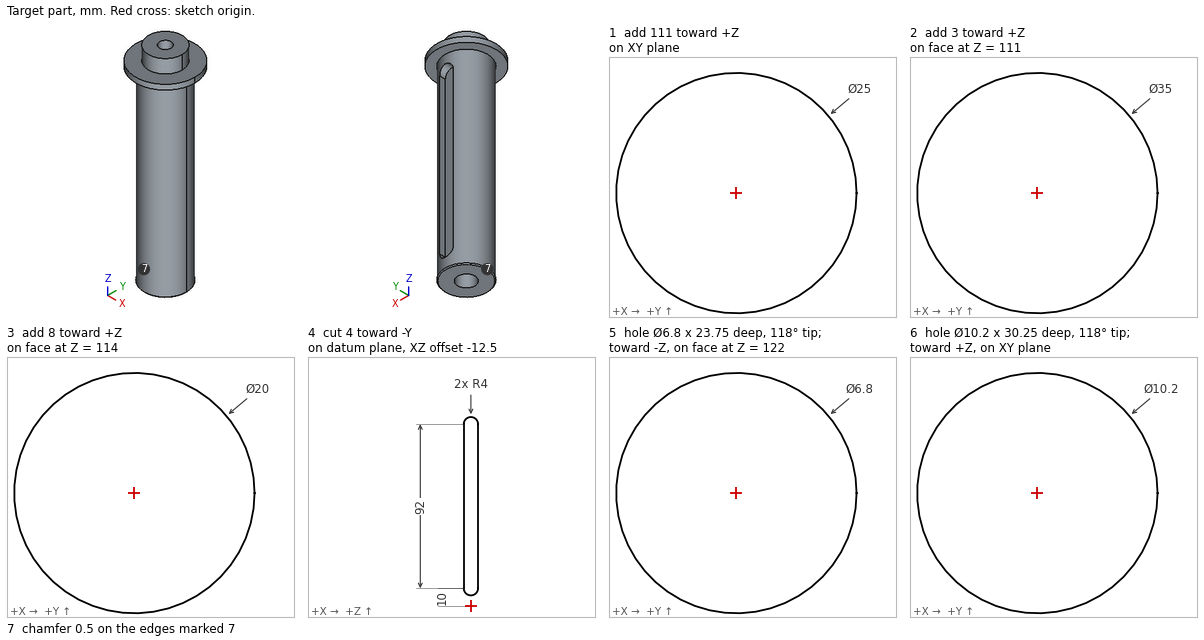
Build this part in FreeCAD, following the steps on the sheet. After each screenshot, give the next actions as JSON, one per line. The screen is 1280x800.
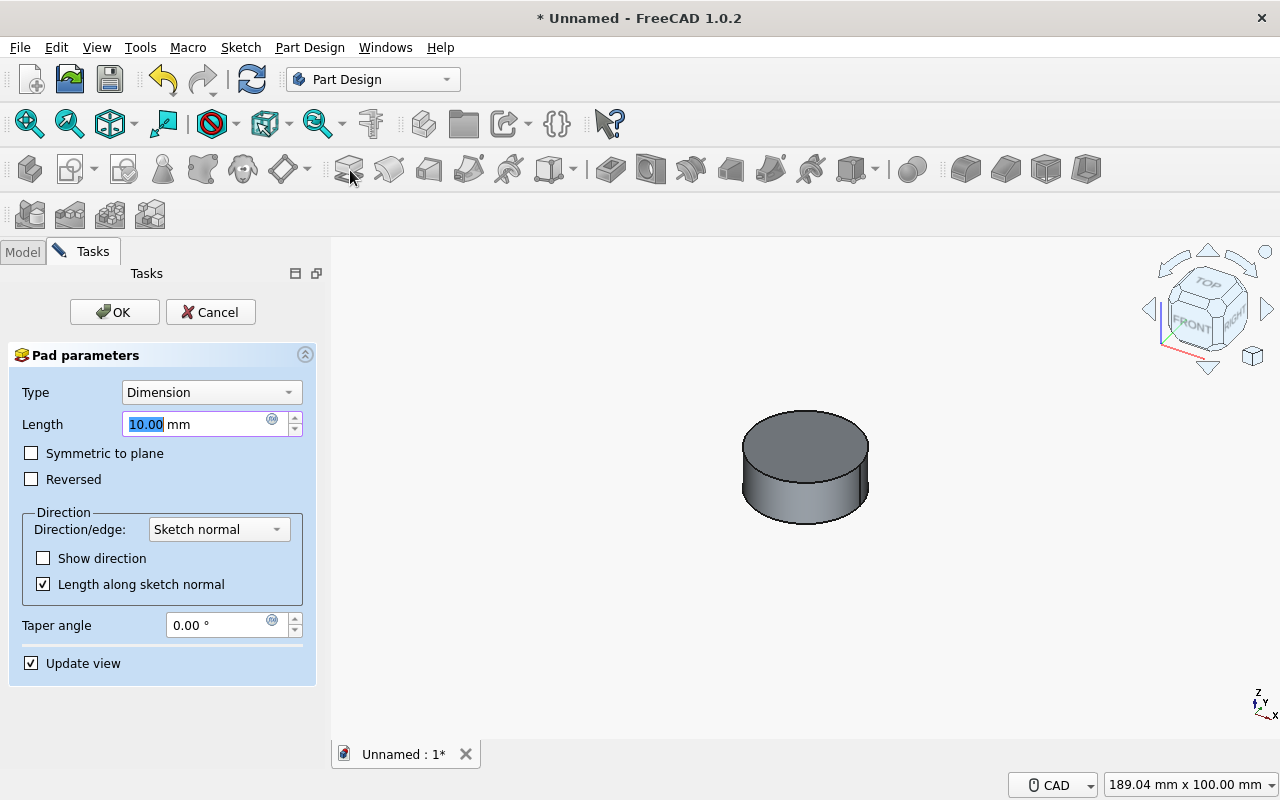
{"action": "type", "text": "111"}
{"action": "key", "text": "Tab"}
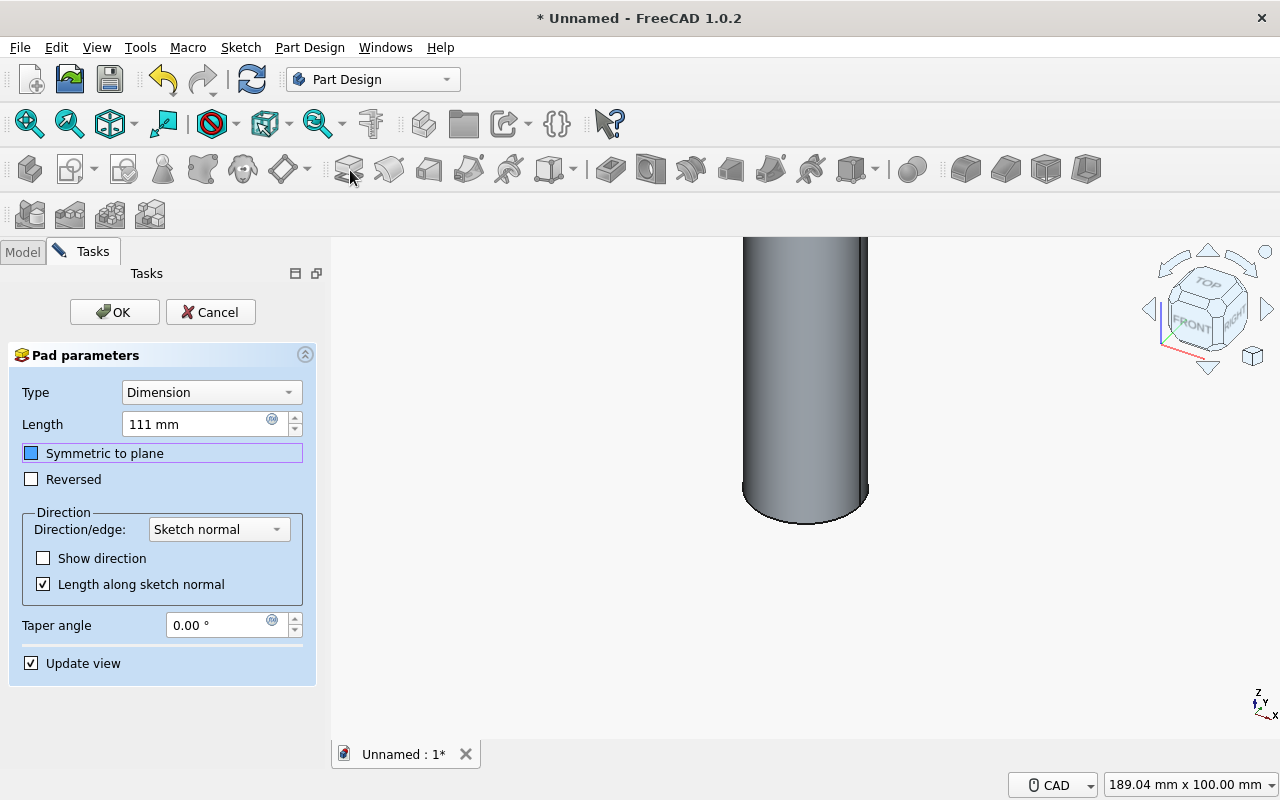
{"action": "left_click", "coordinate": [115, 312]}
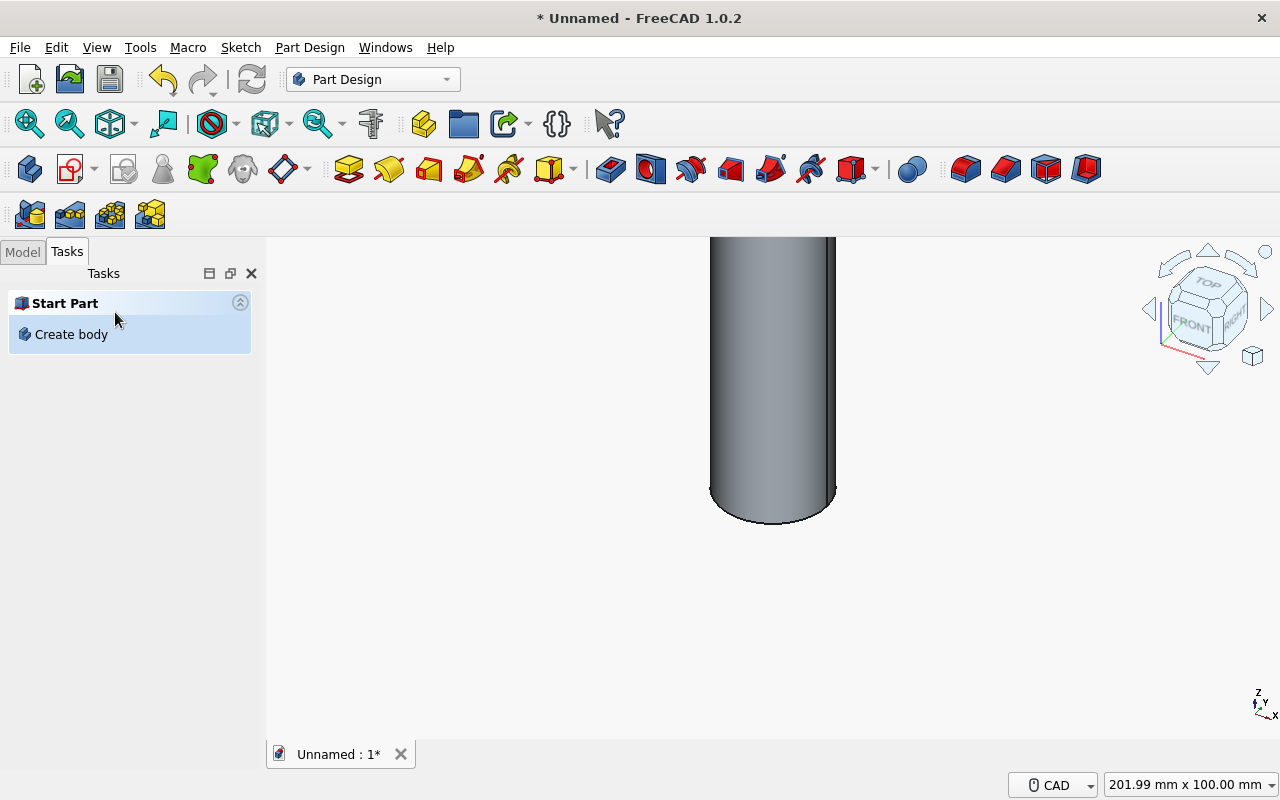
{"action": "key", "text": "v f"}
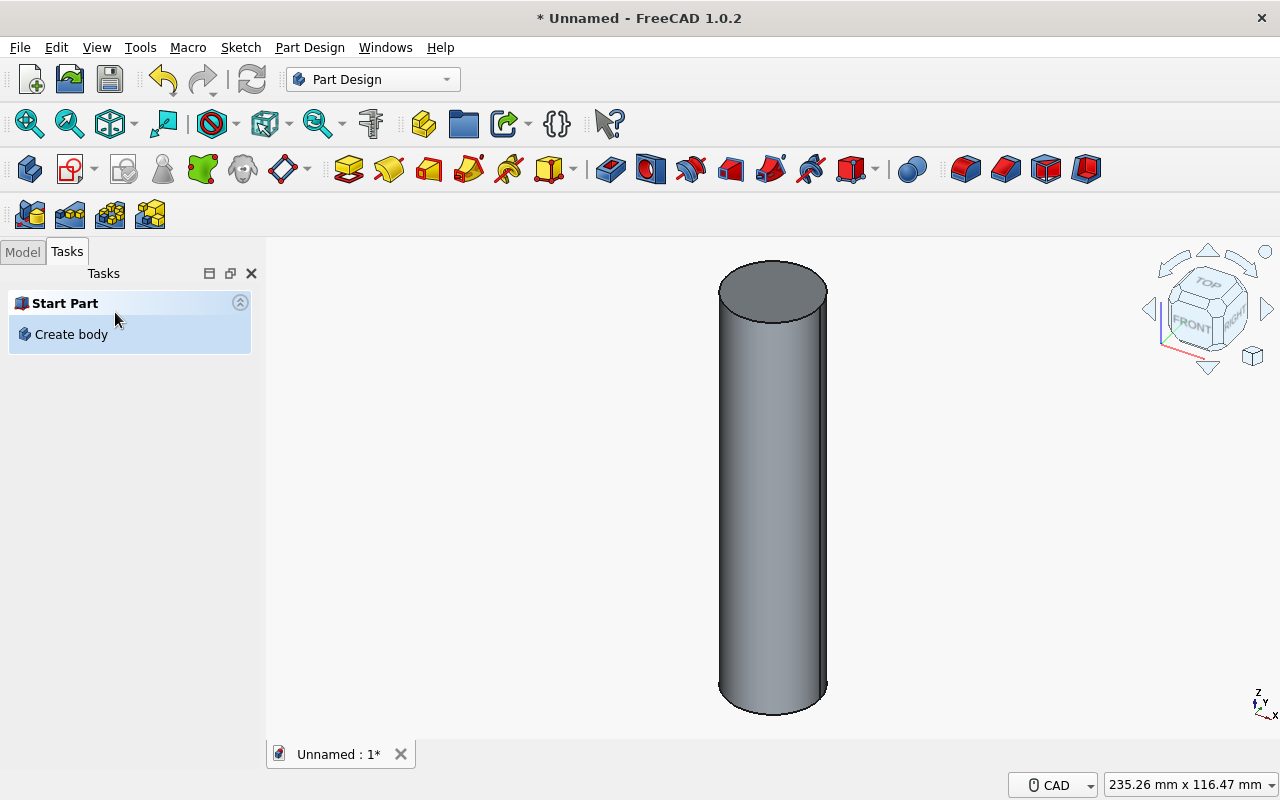
{"action": "left_click", "coordinate": [773, 291]}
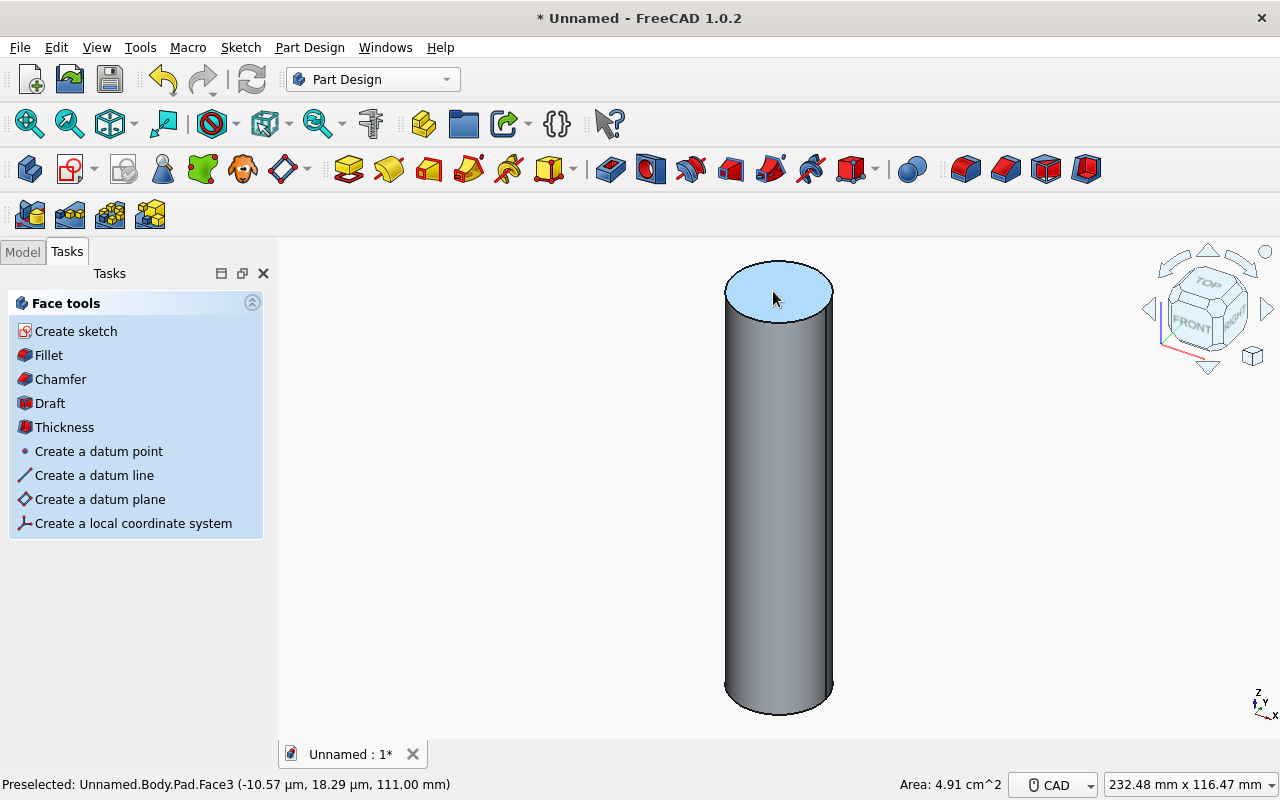
{"action": "left_click", "coordinate": [70, 170]}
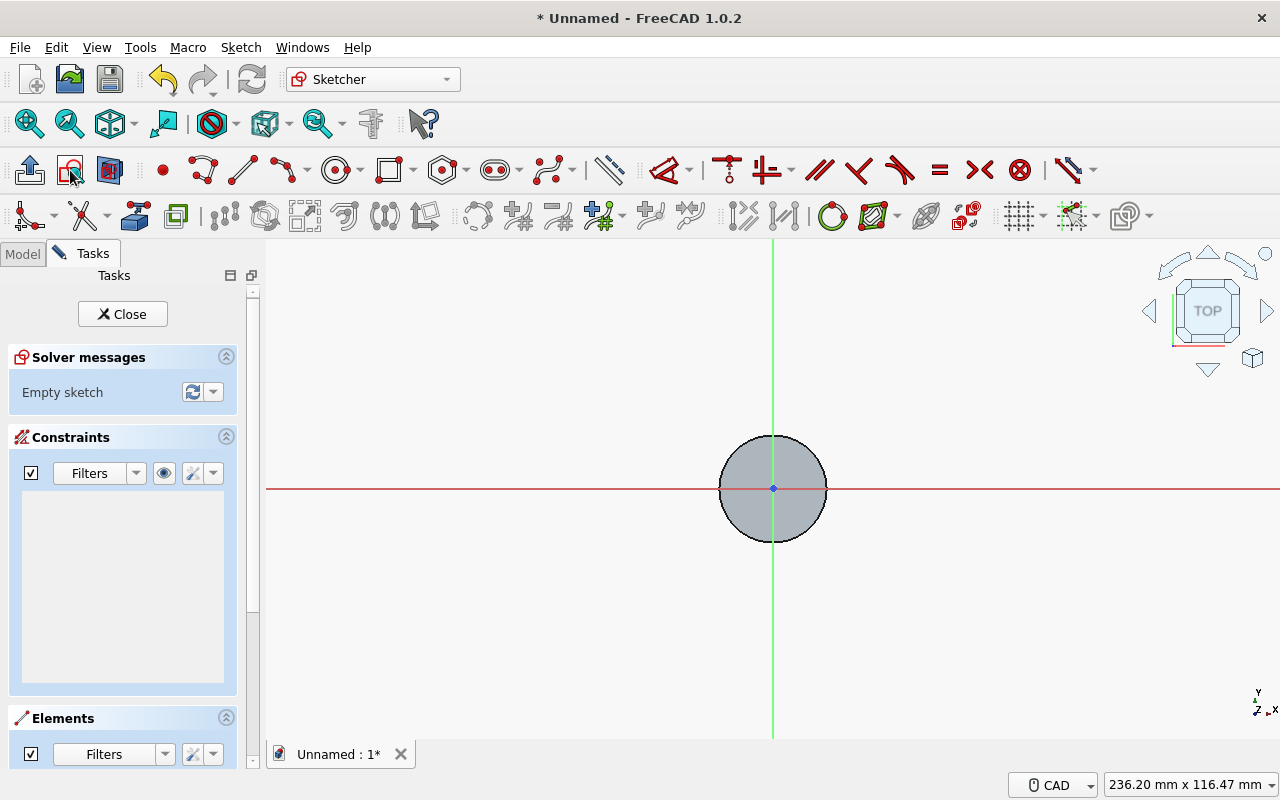
{"action": "scroll", "coordinate": [829, 489], "scroll_direction": "up", "scroll_amount": 4}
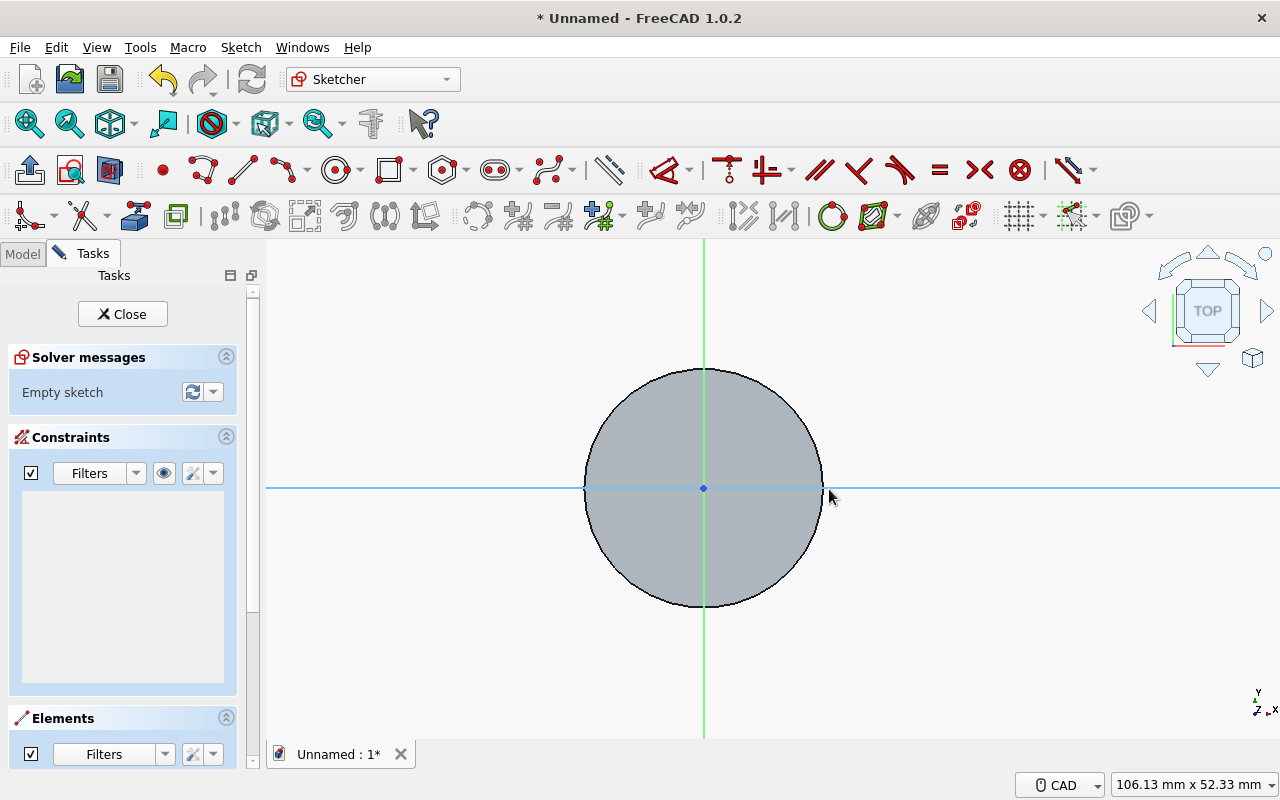
{"action": "key", "text": "g c"}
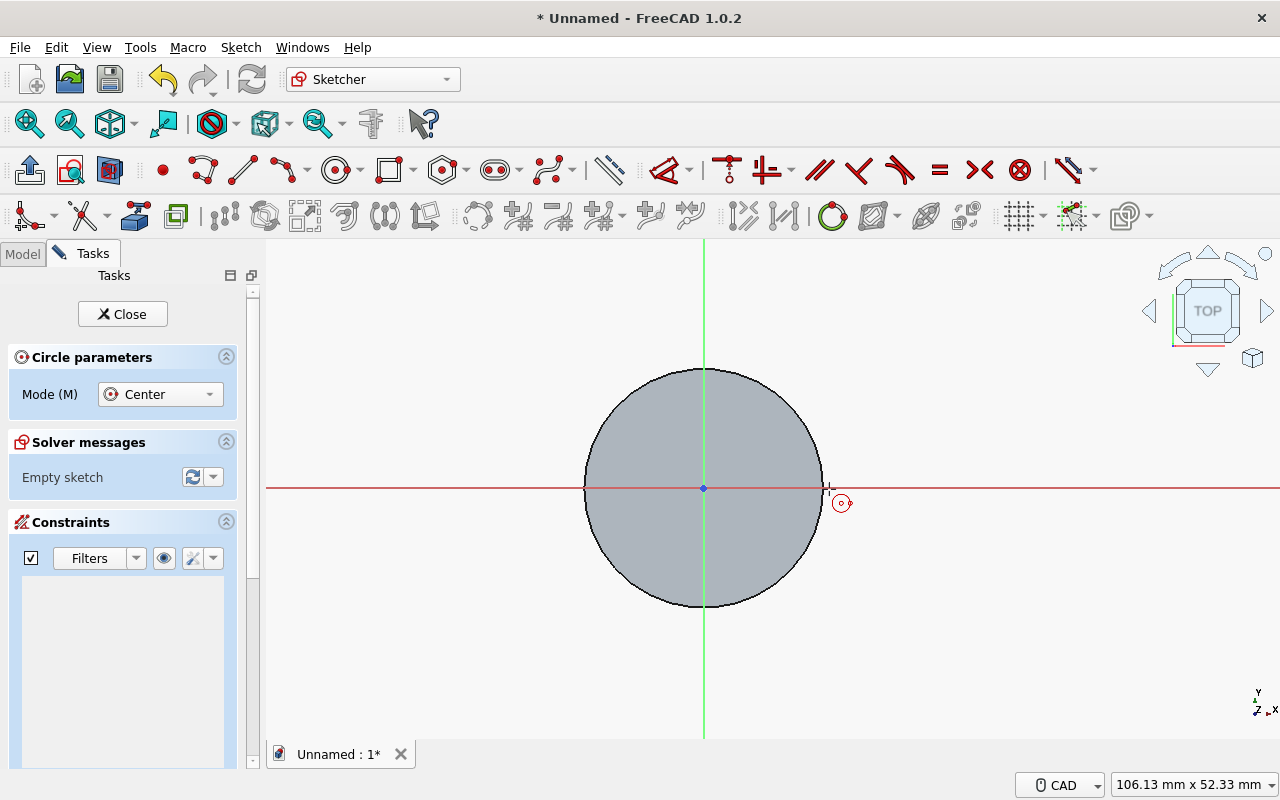
{"action": "left_click", "coordinate": [704, 488]}
{"action": "mouse_move", "coordinate": [822, 370]}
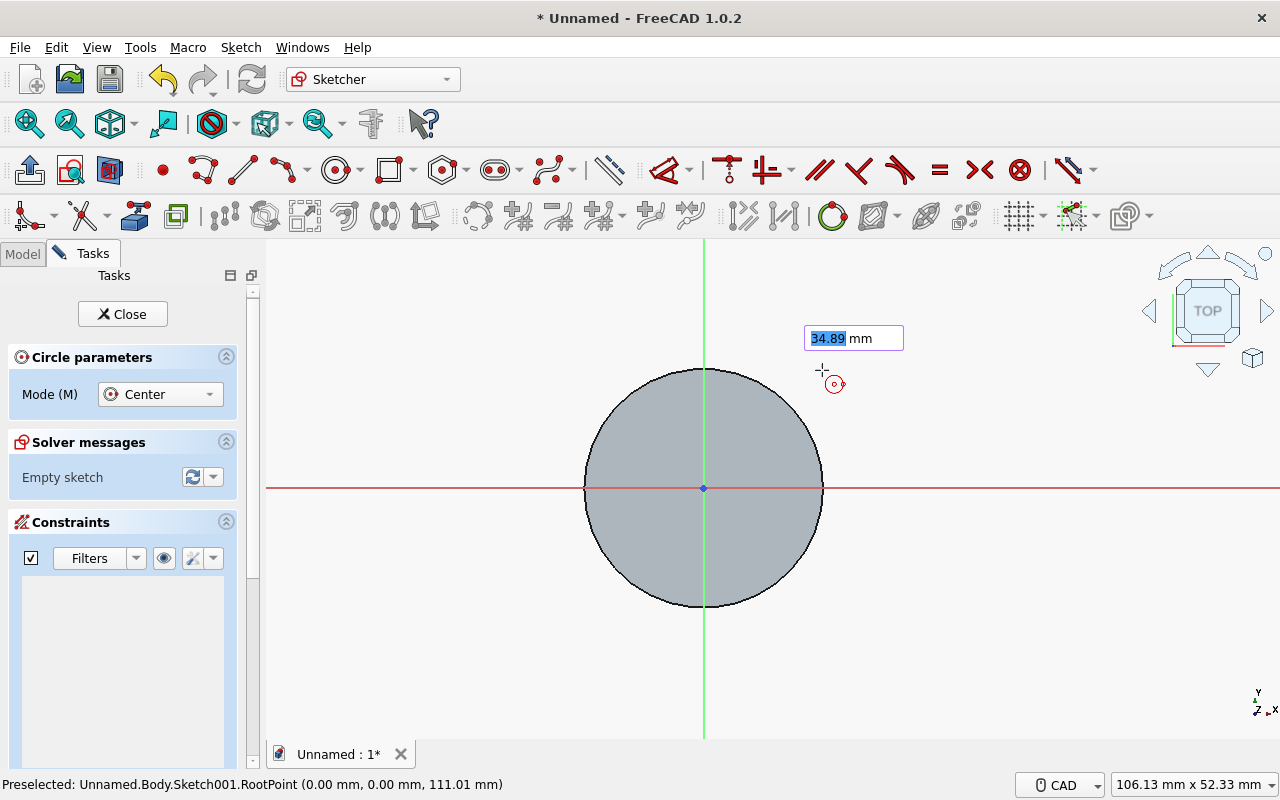
{"action": "type", "text": "35"}
{"action": "key", "text": "Return"}
{"action": "key", "text": "Escape"}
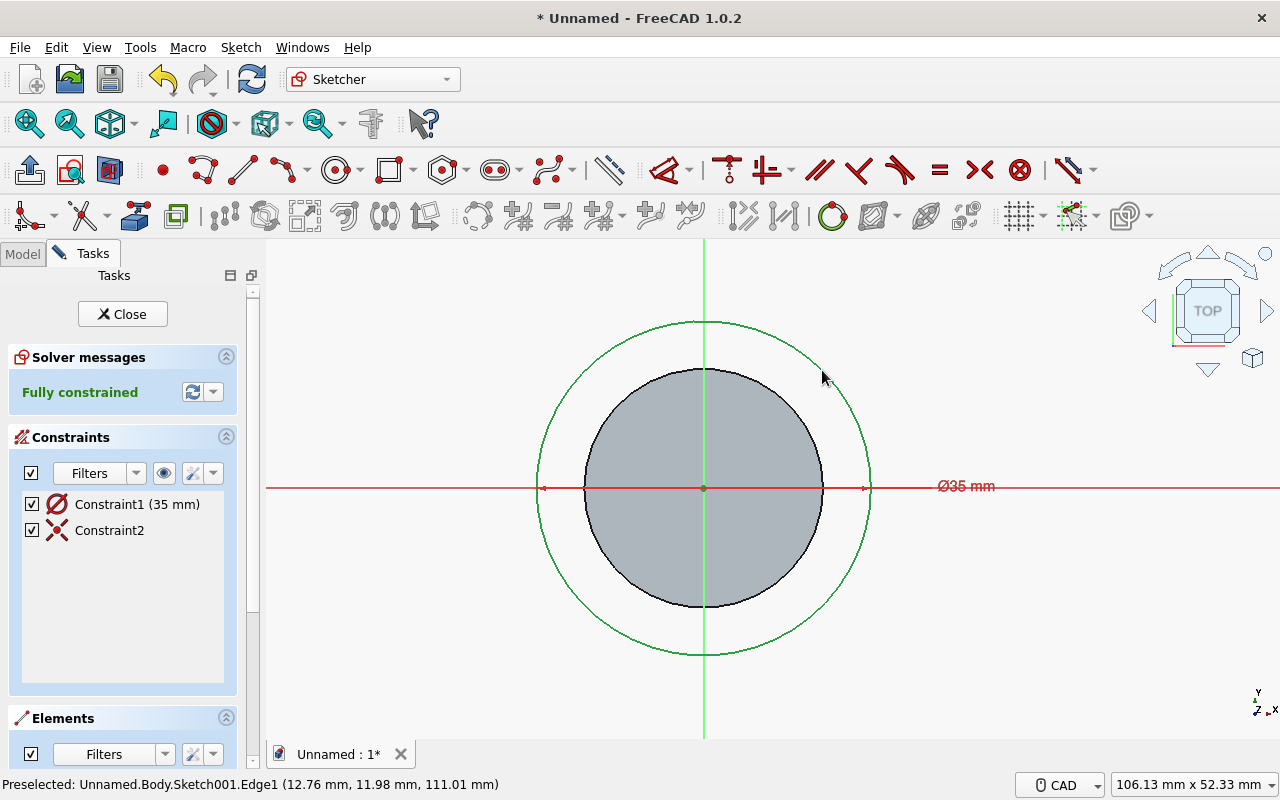
{"action": "left_click", "coordinate": [123, 314]}